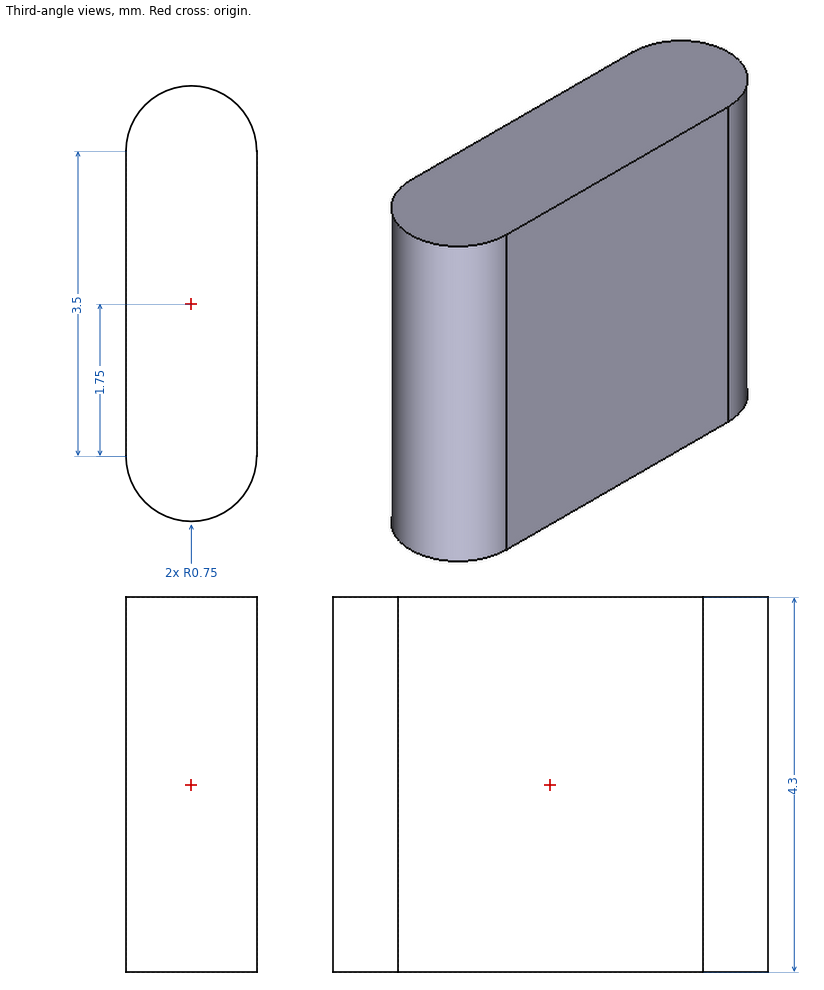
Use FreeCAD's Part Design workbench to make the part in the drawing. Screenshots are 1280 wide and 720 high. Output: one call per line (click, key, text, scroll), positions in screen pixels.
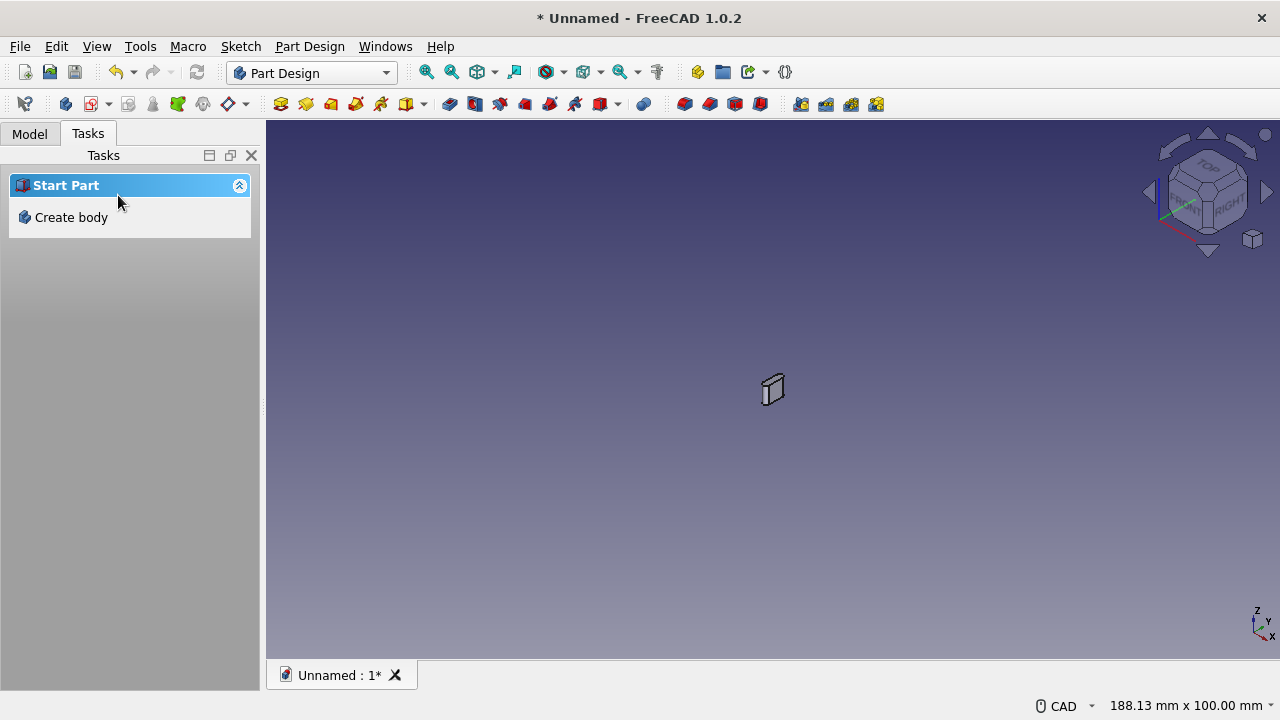
click(427, 72)